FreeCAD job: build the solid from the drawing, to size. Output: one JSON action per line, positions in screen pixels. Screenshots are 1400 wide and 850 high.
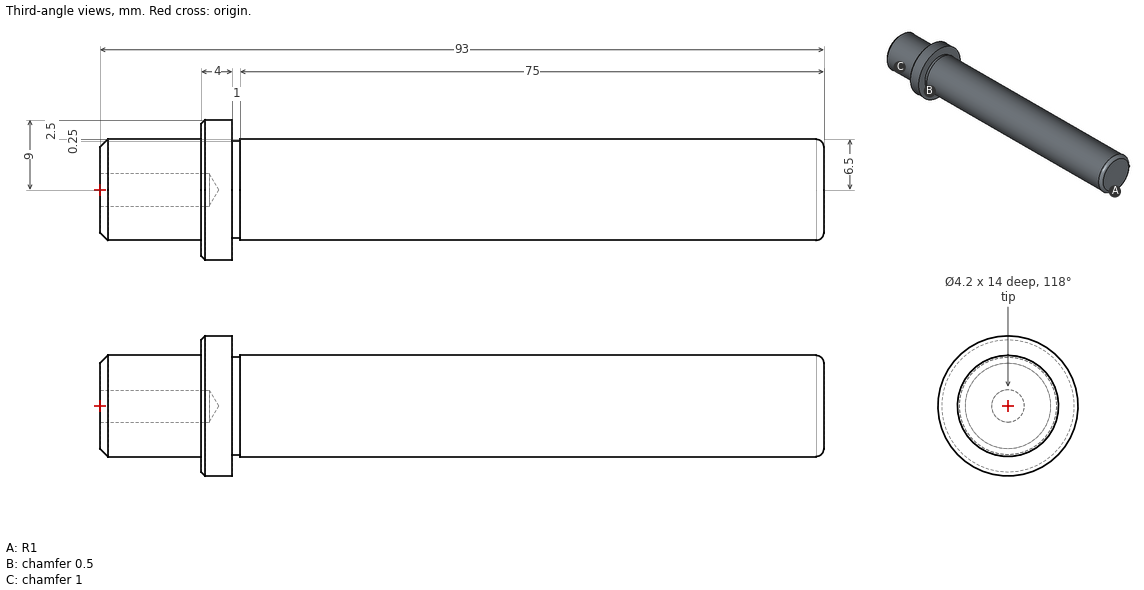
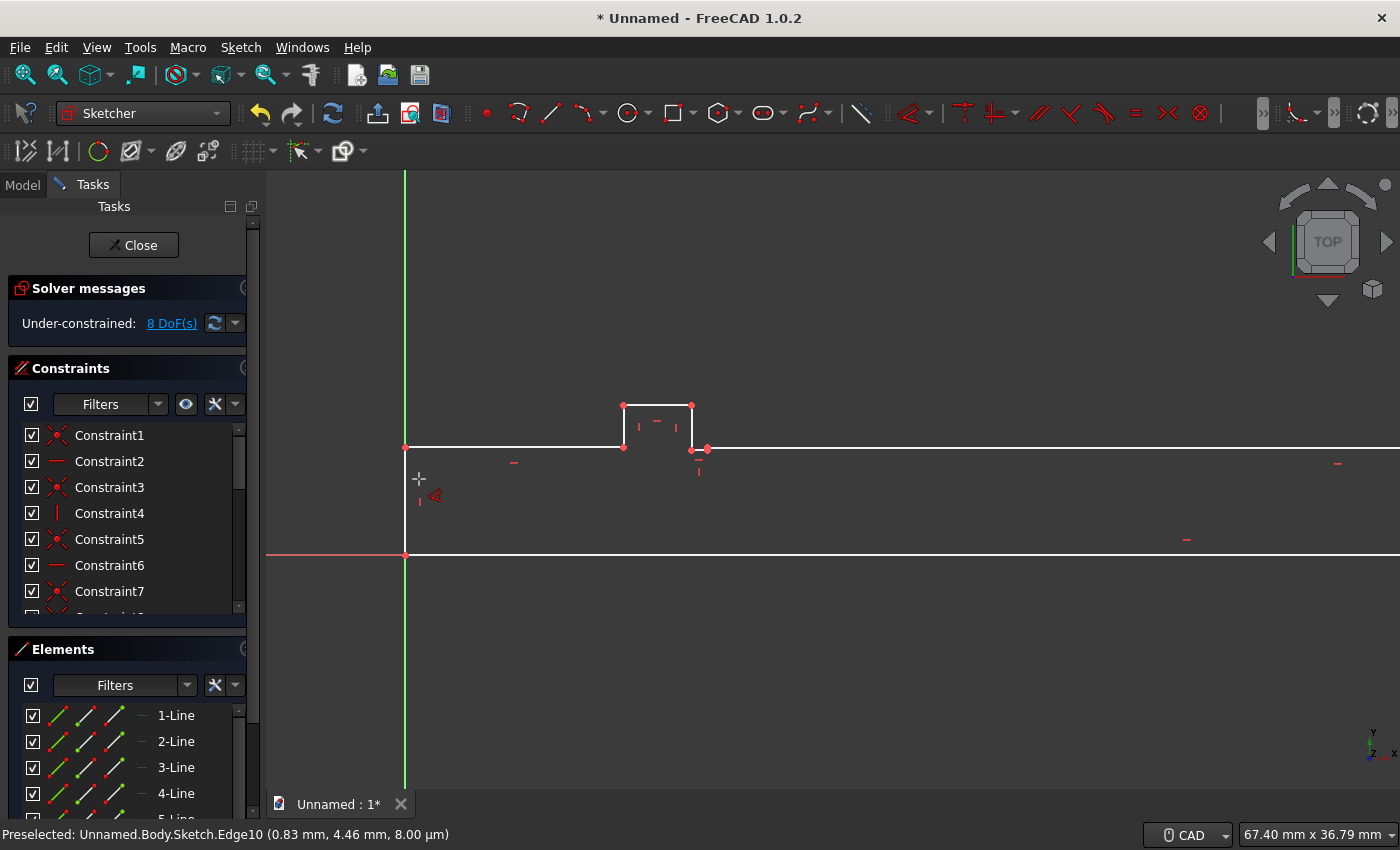
{"action": "scroll", "coordinate": [700, 450], "scroll_direction": "up", "scroll_amount": 5}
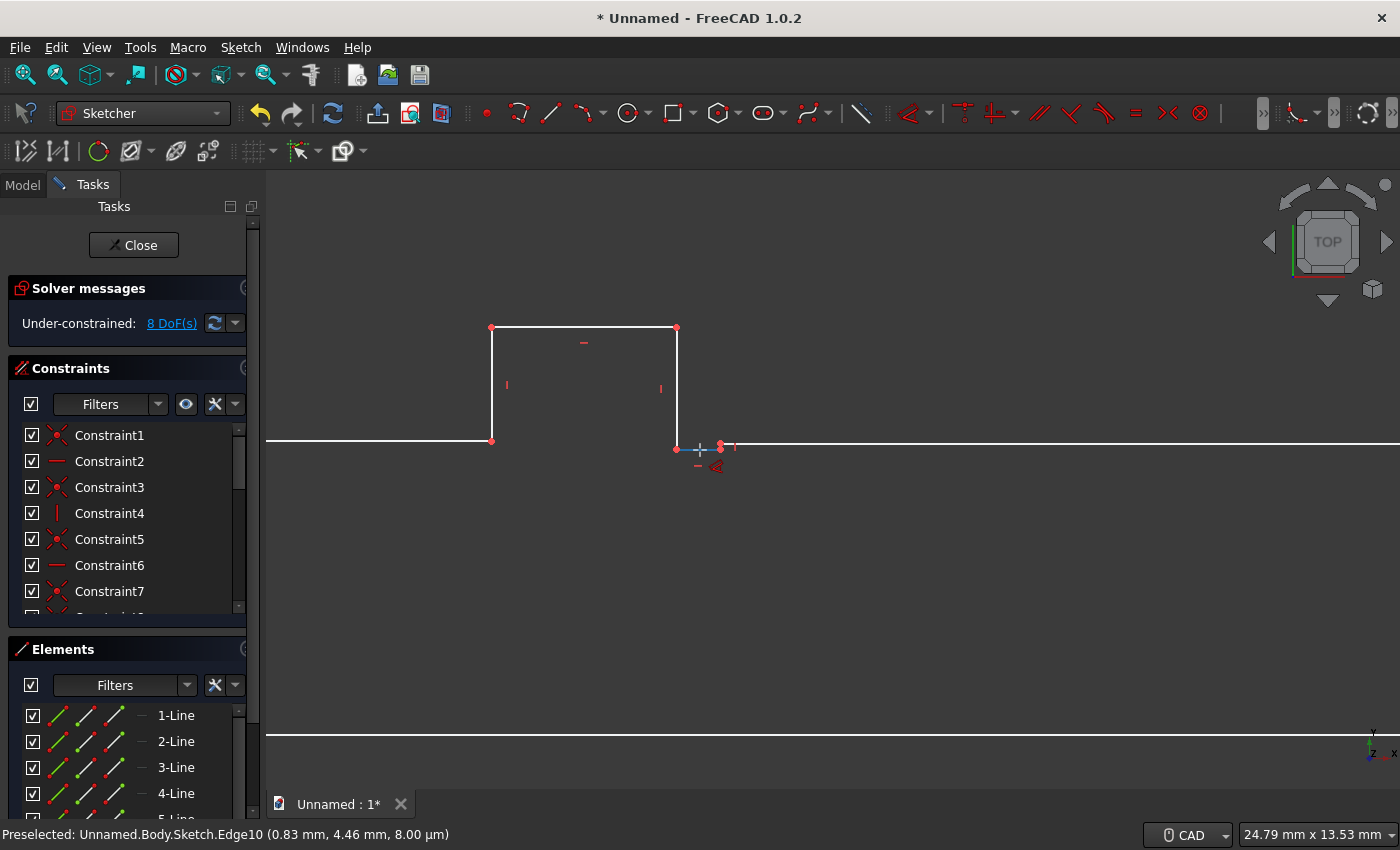
{"action": "left_click", "coordinate": [698, 450]}
{"action": "left_click", "coordinate": [698, 416]}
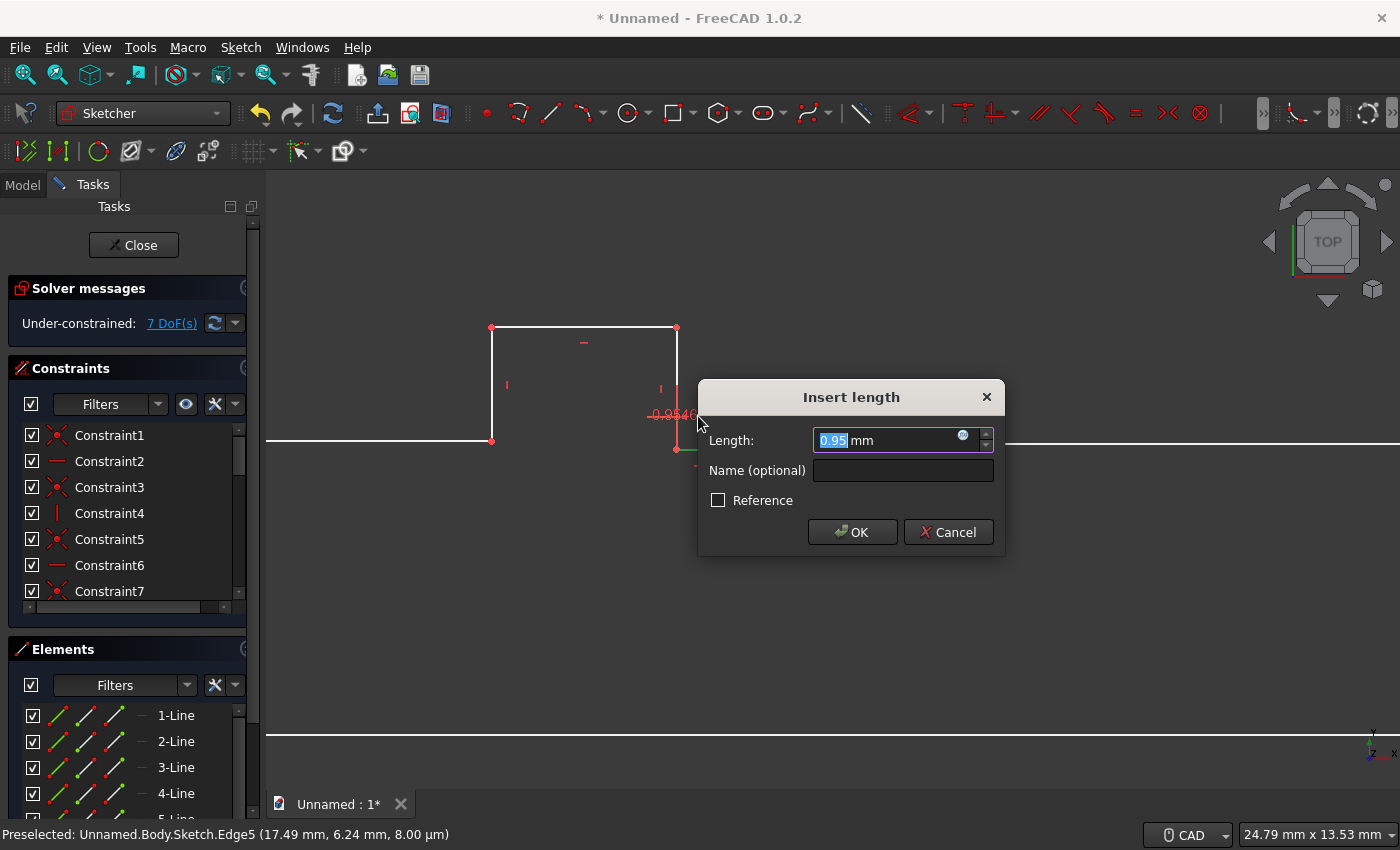
{"action": "type", "text": "1"}
{"action": "key", "text": "Return"}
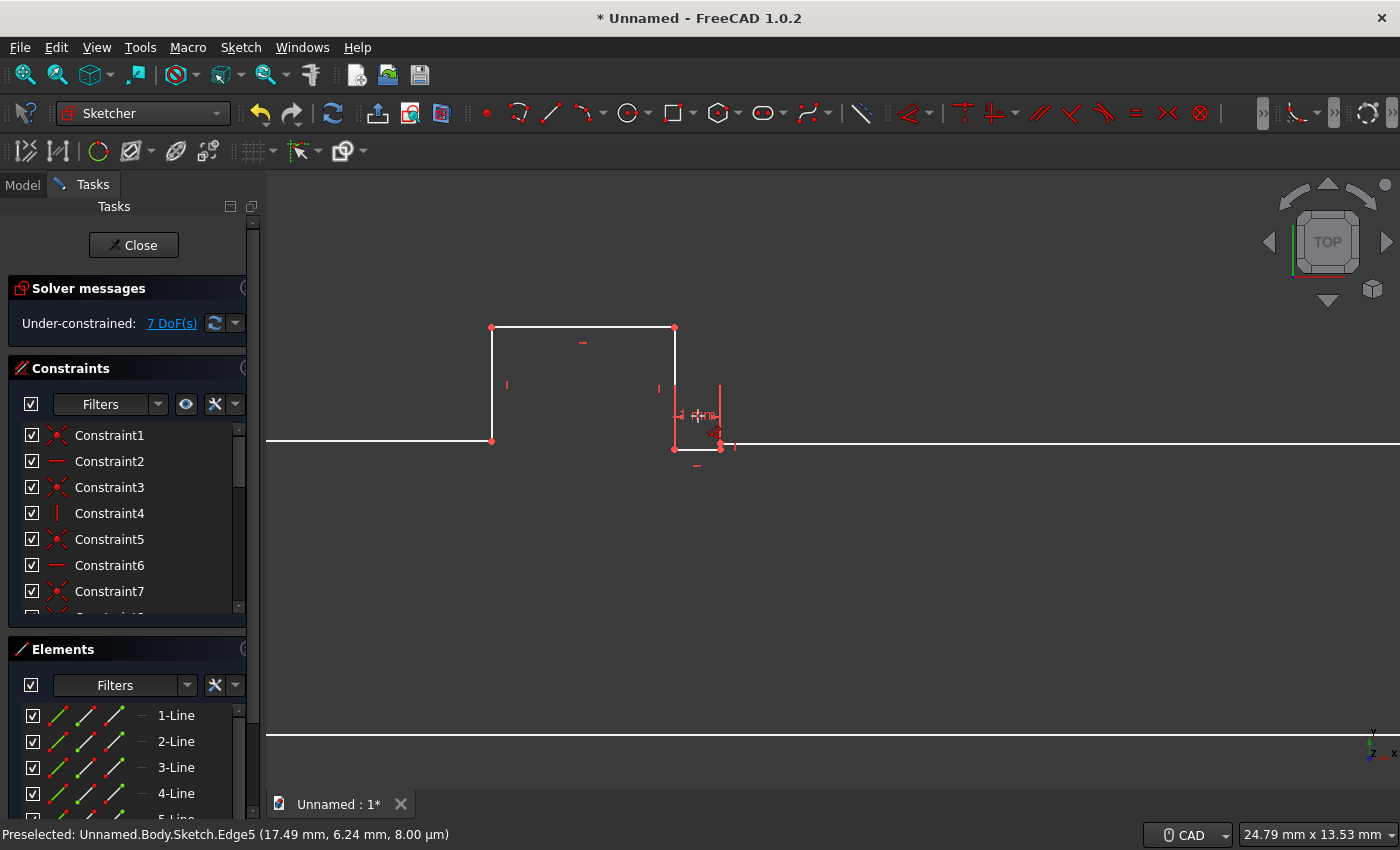
{"action": "scroll", "coordinate": [515, 470], "scroll_direction": "down", "scroll_amount": 9}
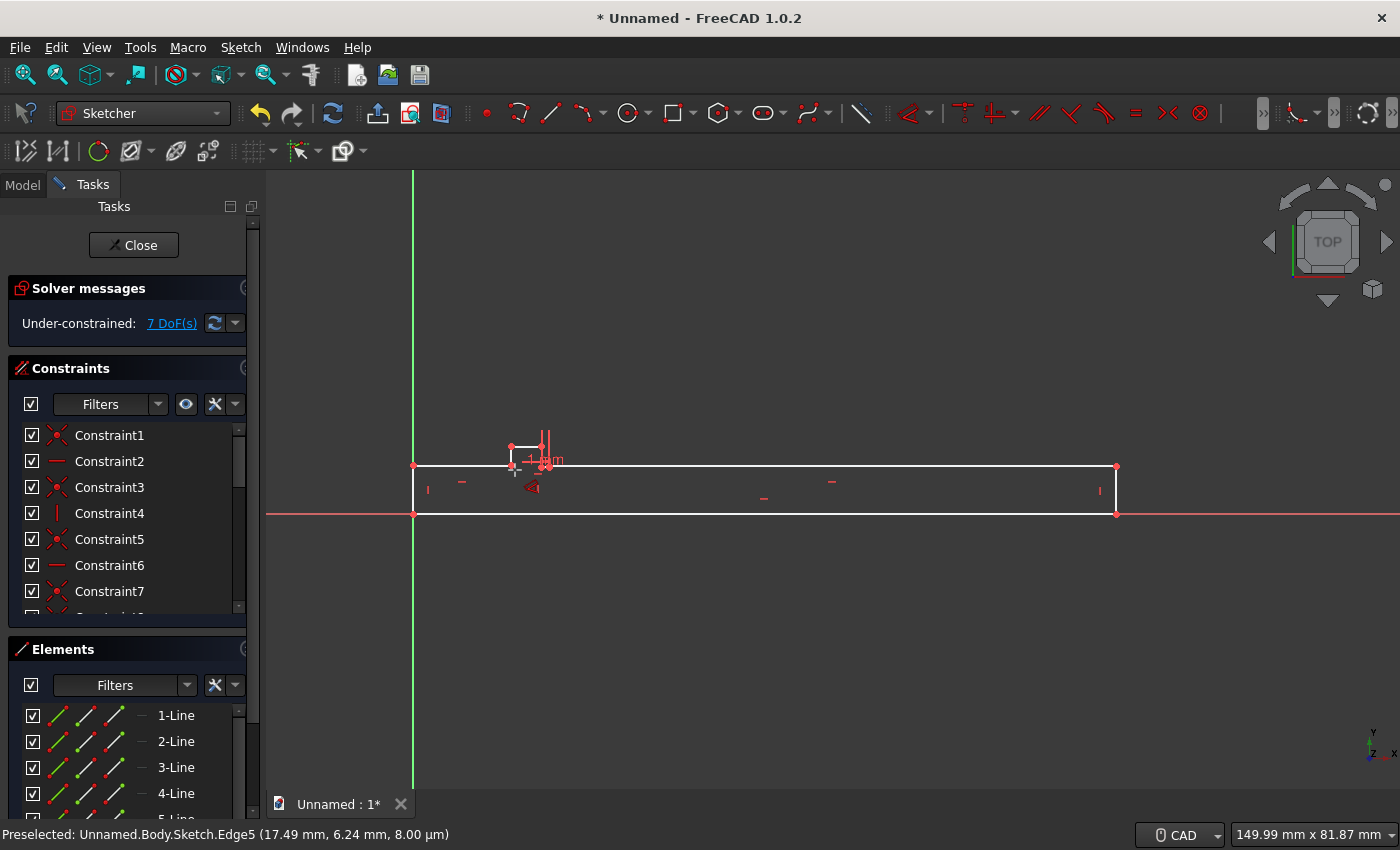
{"action": "scroll", "coordinate": [532, 447], "scroll_direction": "up", "scroll_amount": 3}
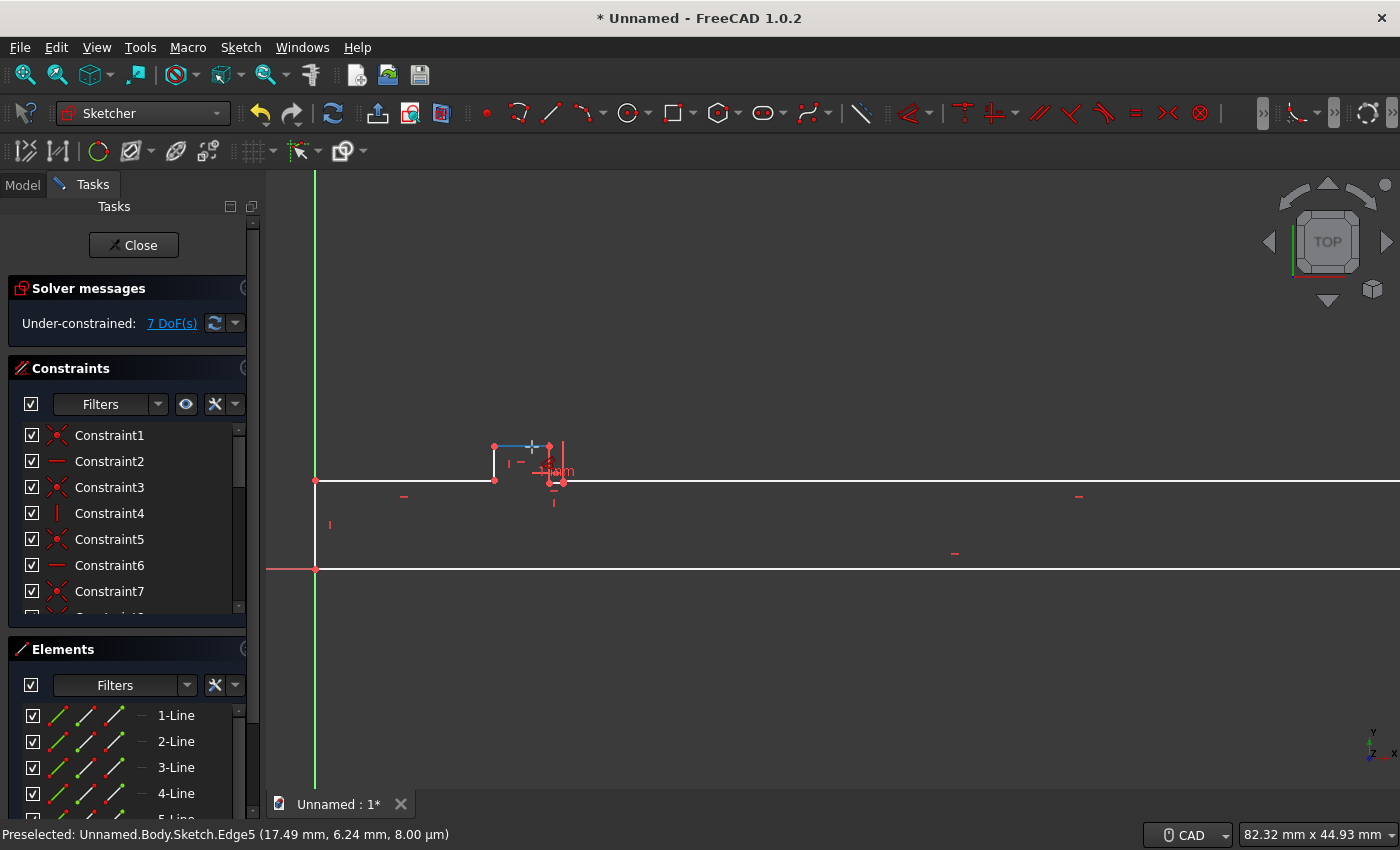
{"action": "left_click", "coordinate": [533, 446]}
{"action": "left_click", "coordinate": [522, 412]}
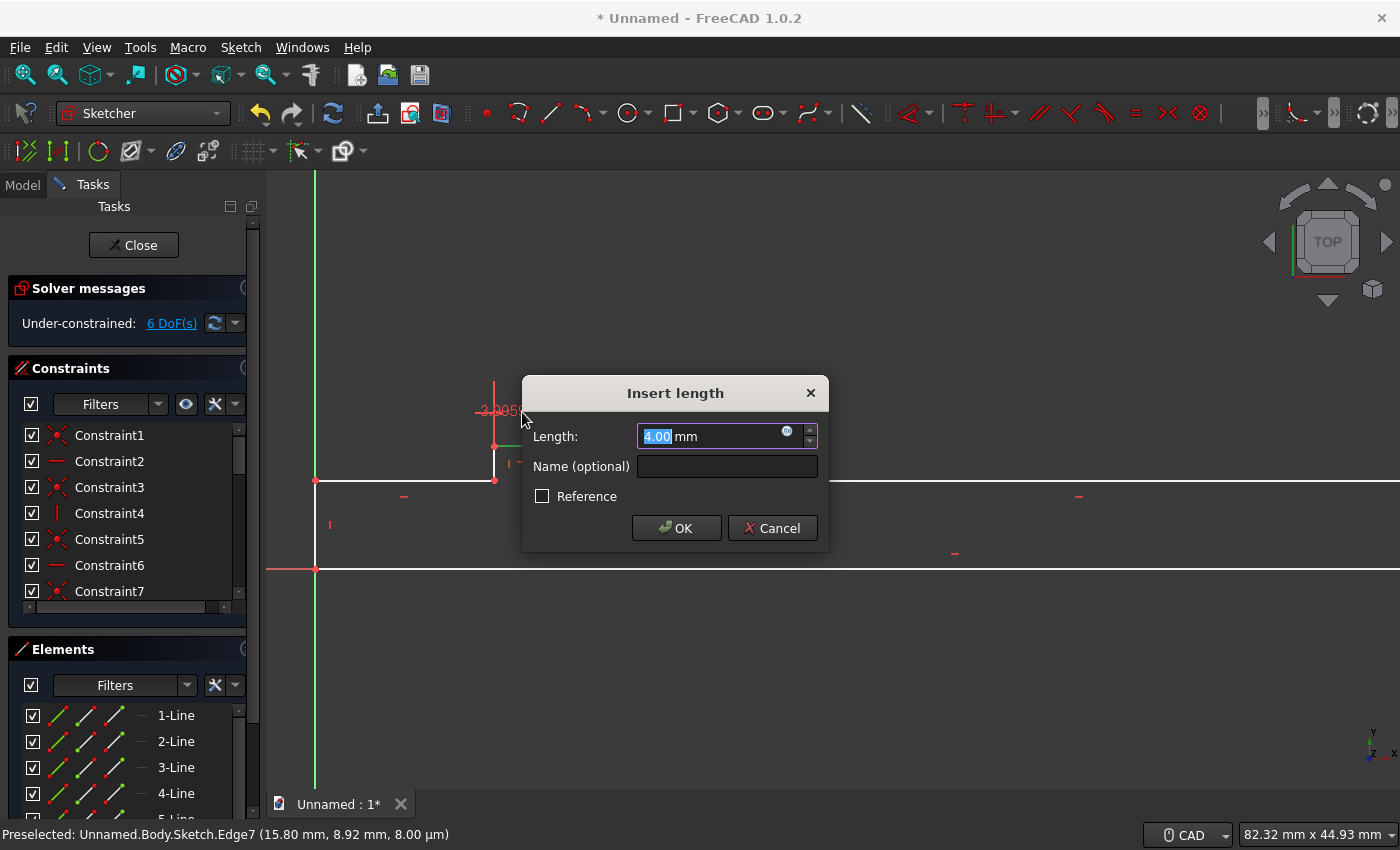
{"action": "type", "text": "4"}
{"action": "key", "text": "Return"}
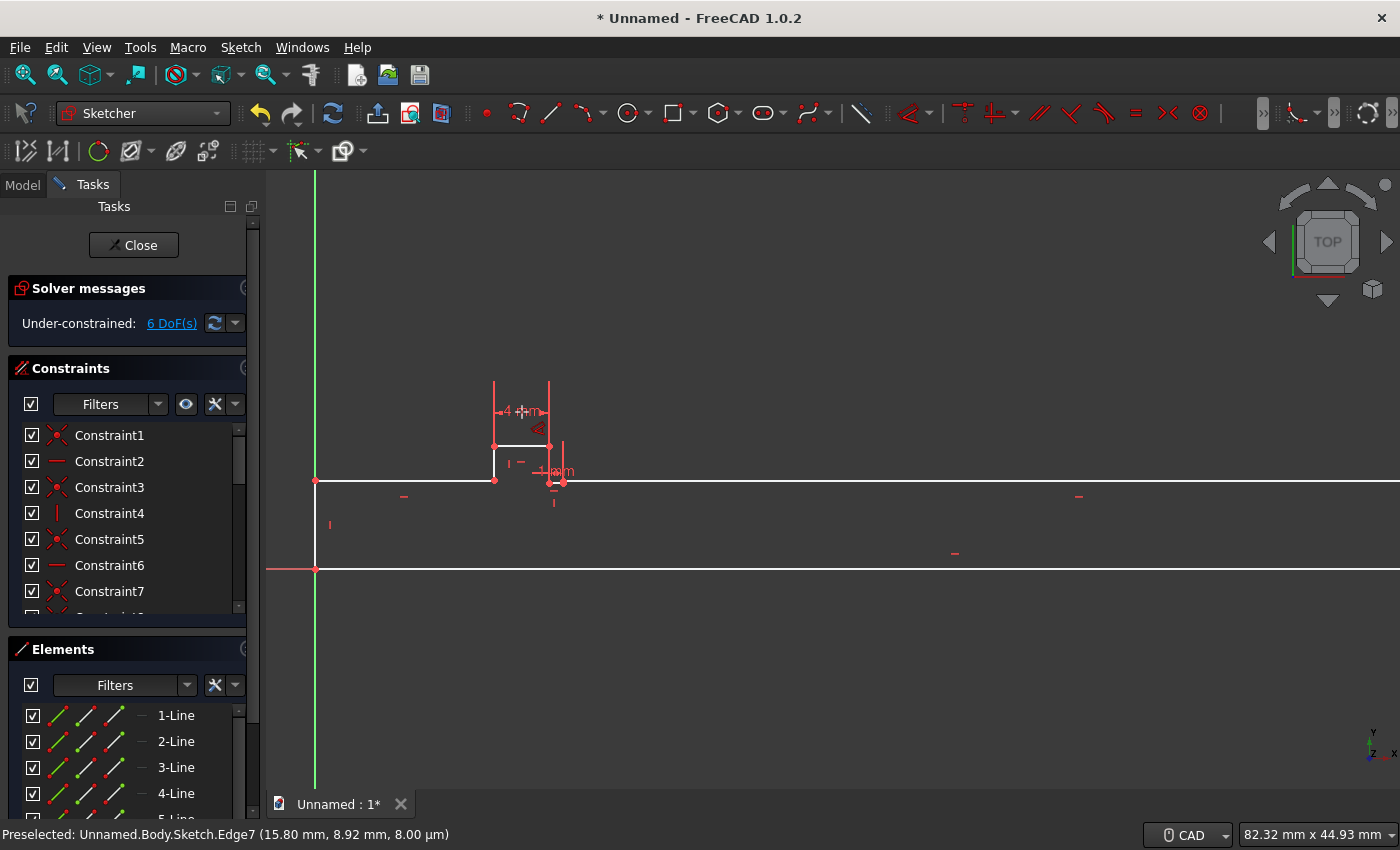
{"action": "left_click", "coordinate": [700, 569]}
{"action": "left_click", "coordinate": [775, 603]}